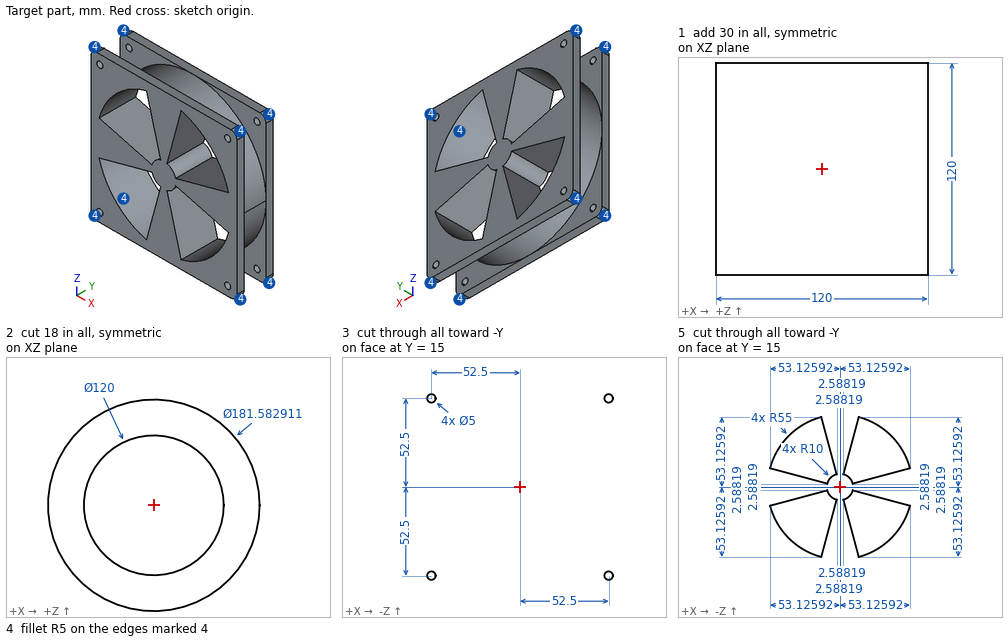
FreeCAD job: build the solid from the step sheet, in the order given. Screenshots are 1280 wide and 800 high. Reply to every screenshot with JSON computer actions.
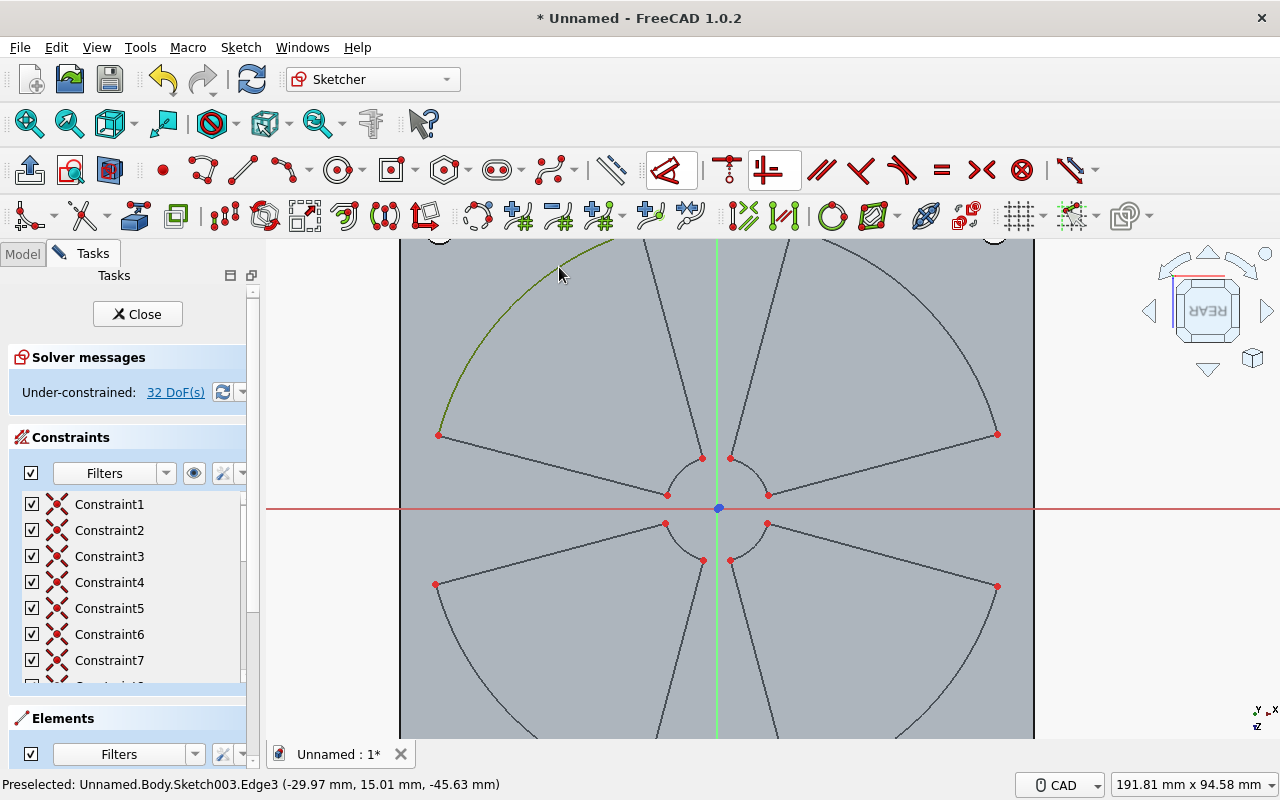
{"action": "left_click", "coordinate": [745, 554]}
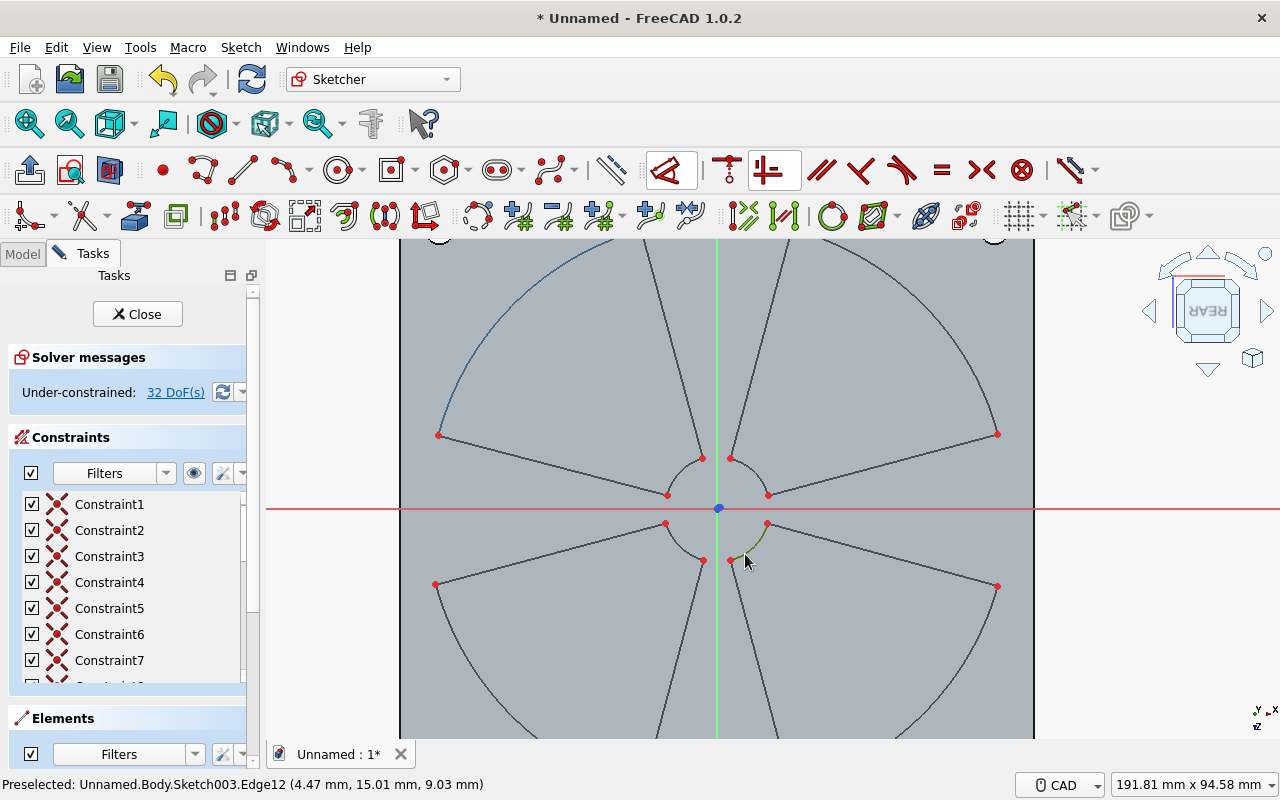
{"action": "left_click", "coordinate": [728, 170]}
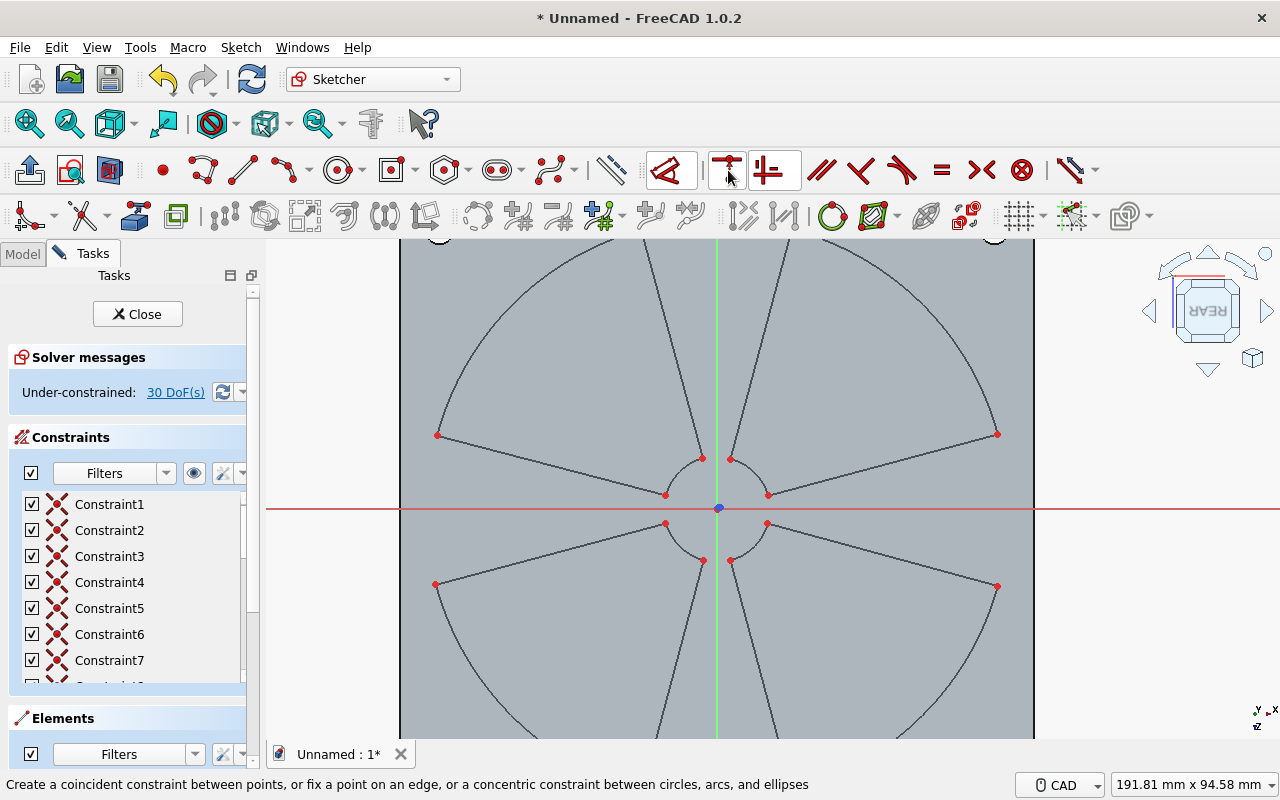
{"action": "left_click", "coordinate": [559, 267]}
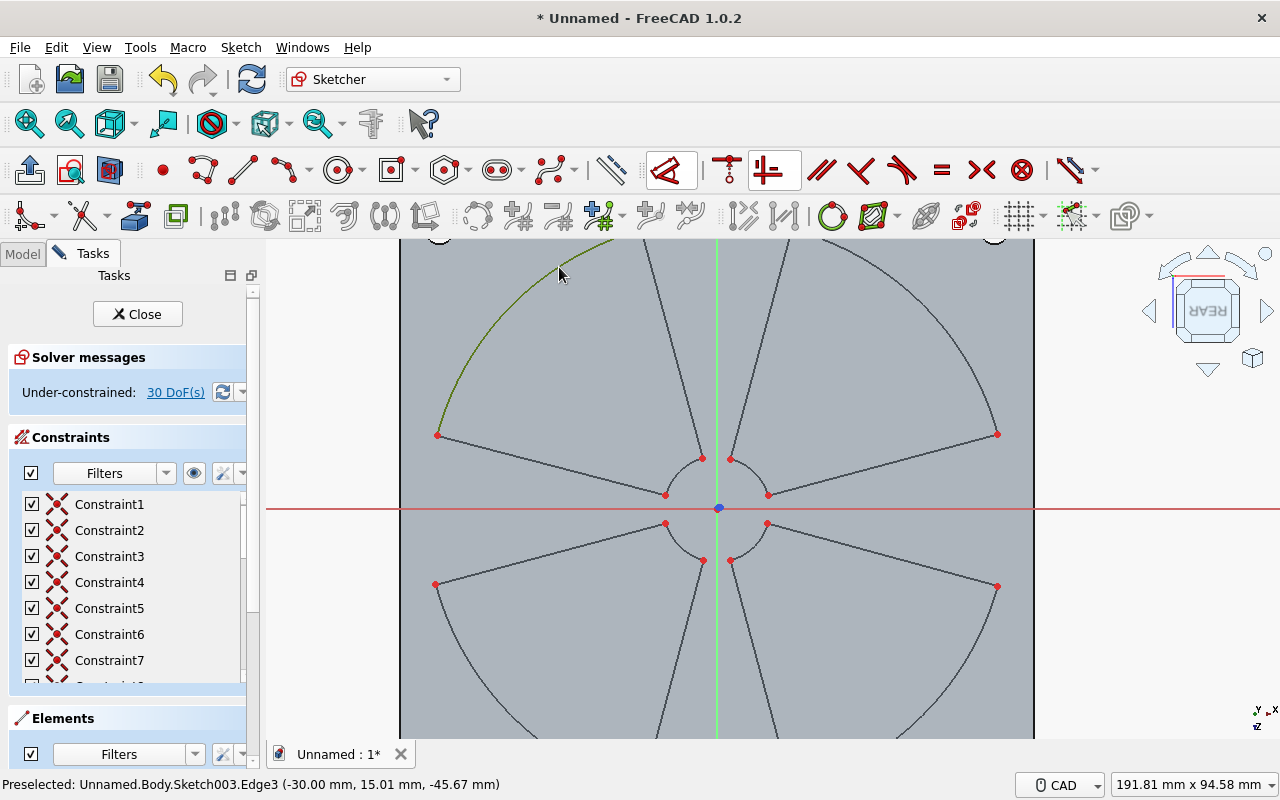
{"action": "left_click", "coordinate": [673, 538]}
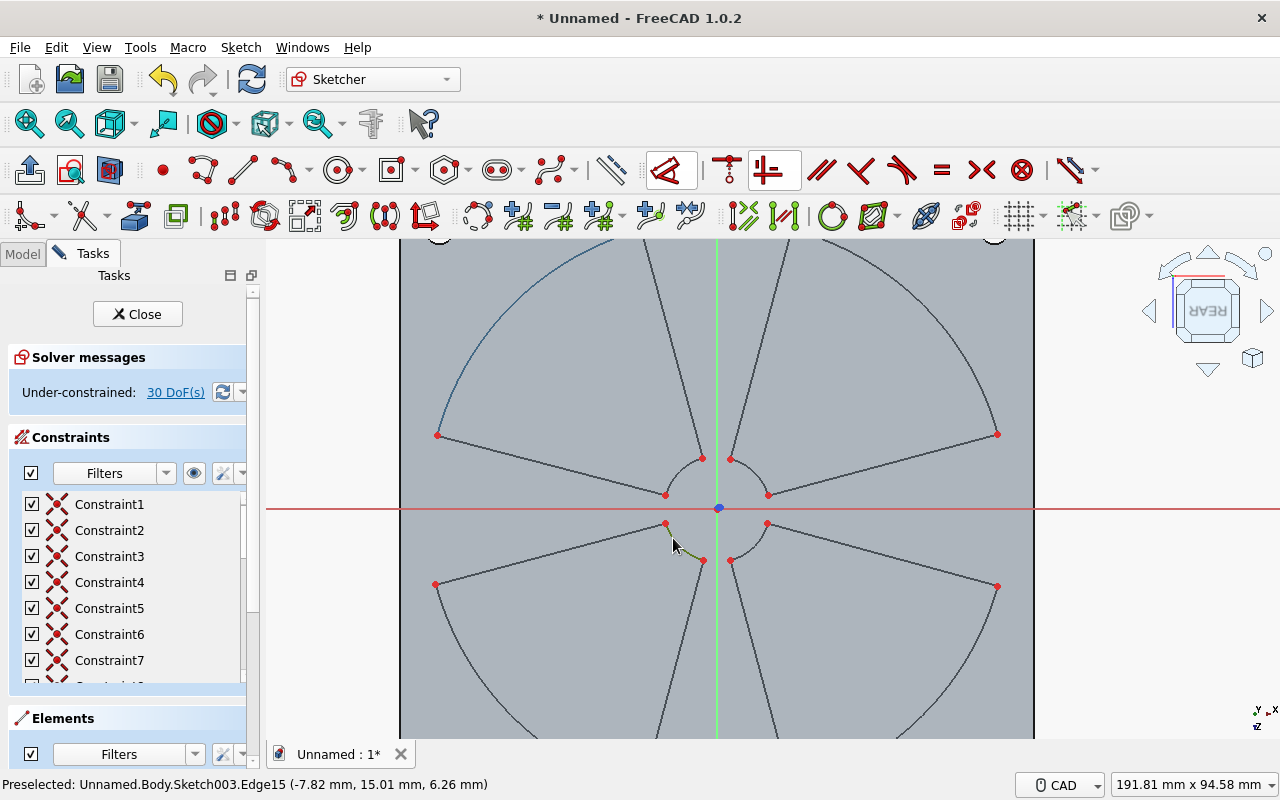
{"action": "left_click", "coordinate": [728, 170]}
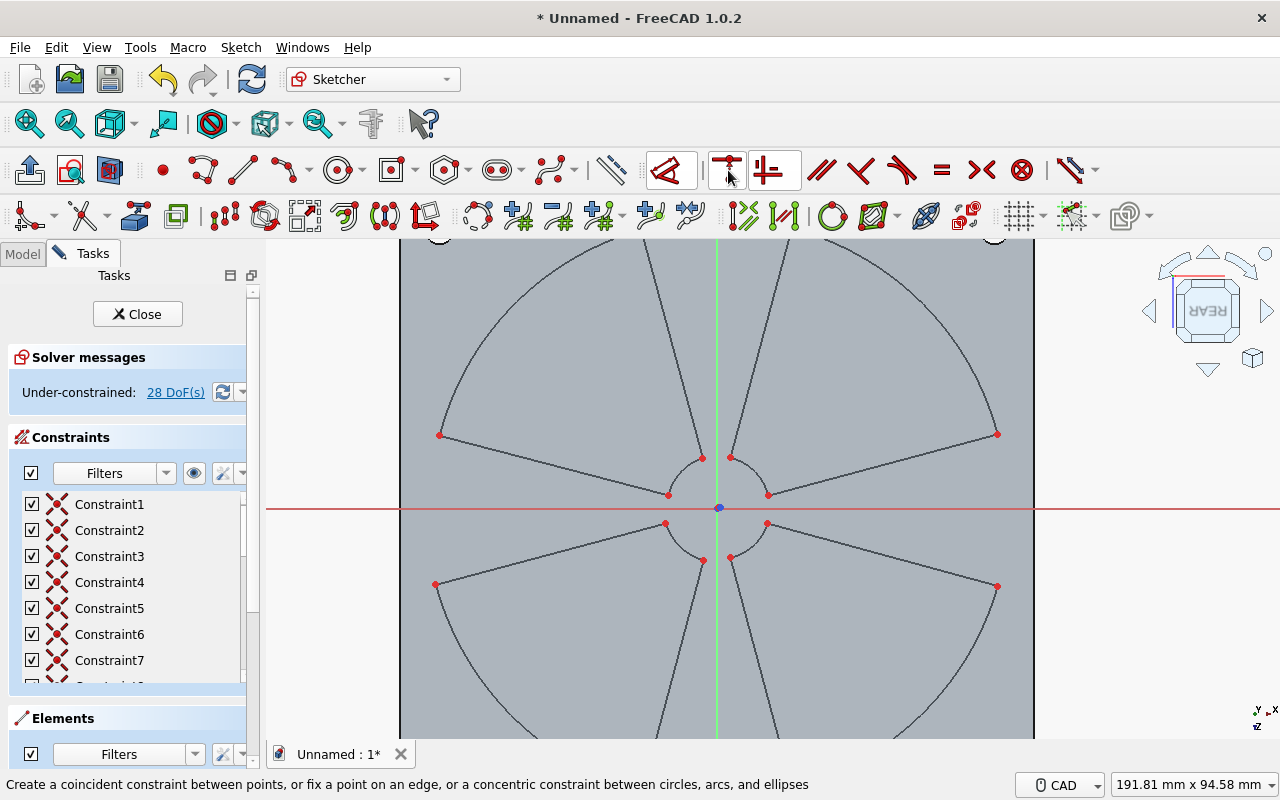
{"action": "left_click", "coordinate": [559, 267]}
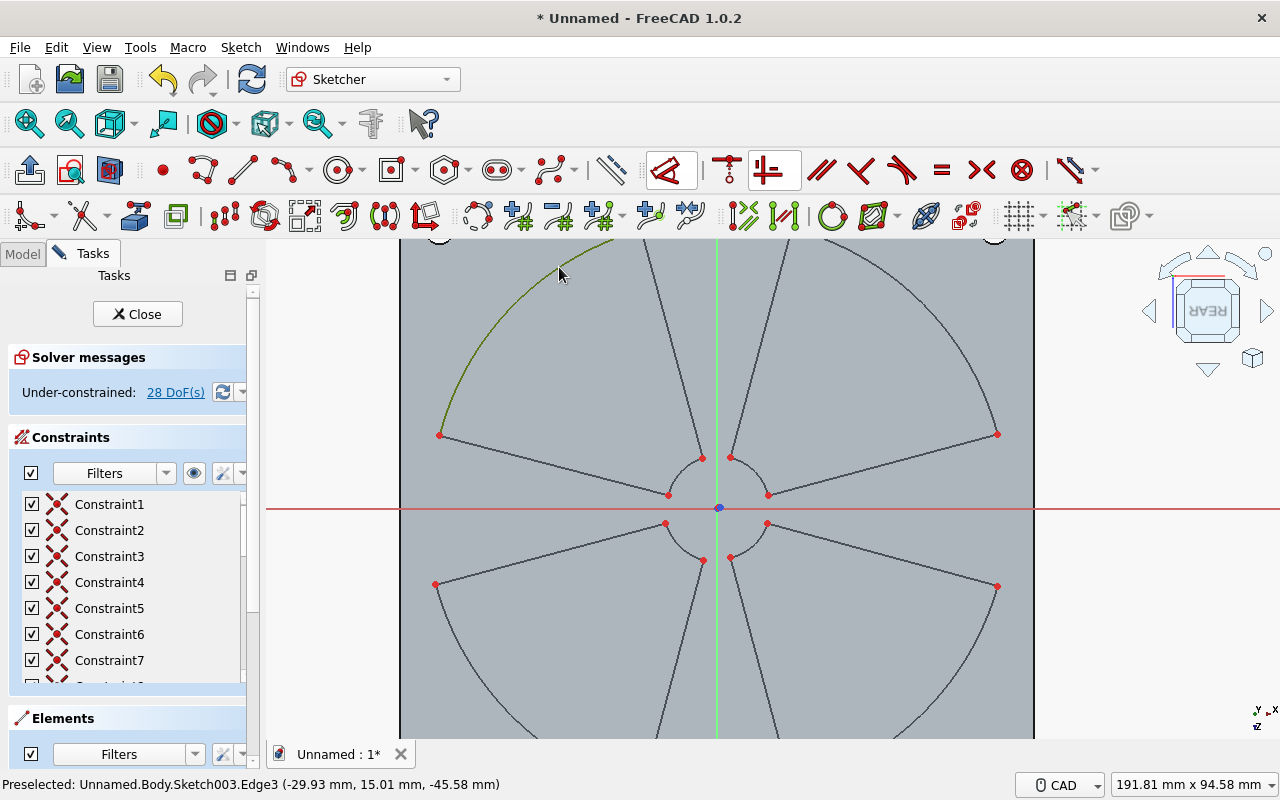
{"action": "left_click", "coordinate": [473, 668]}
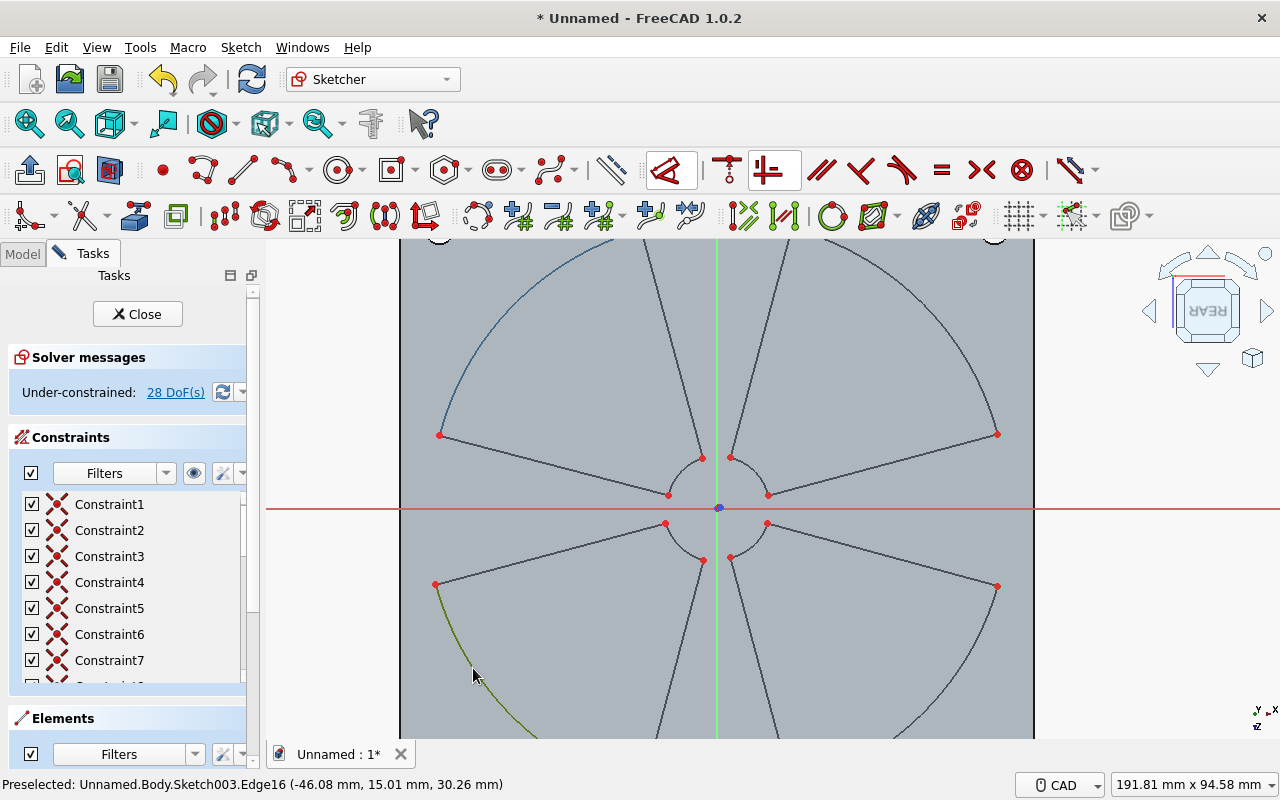
{"action": "left_click", "coordinate": [728, 170]}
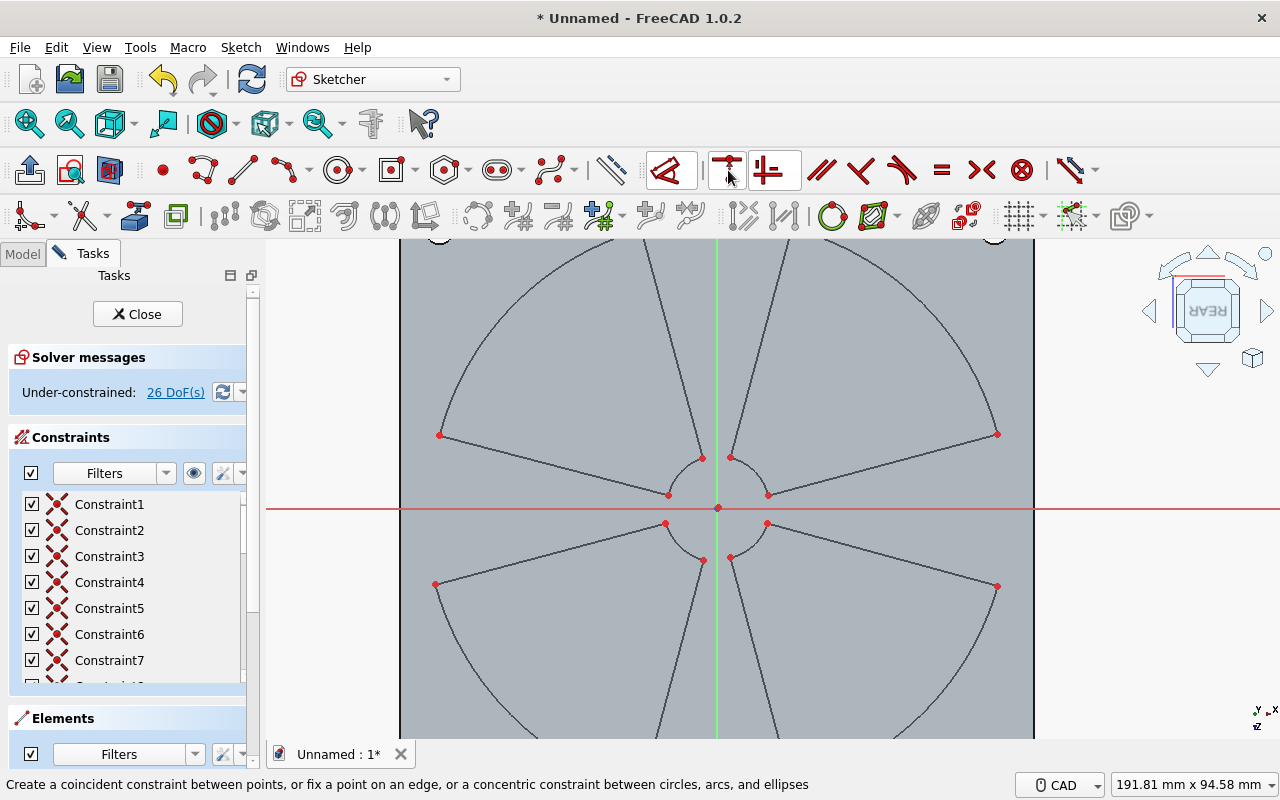
{"action": "left_click_drag", "start_coordinate": [707, 497], "coordinate": [729, 519]}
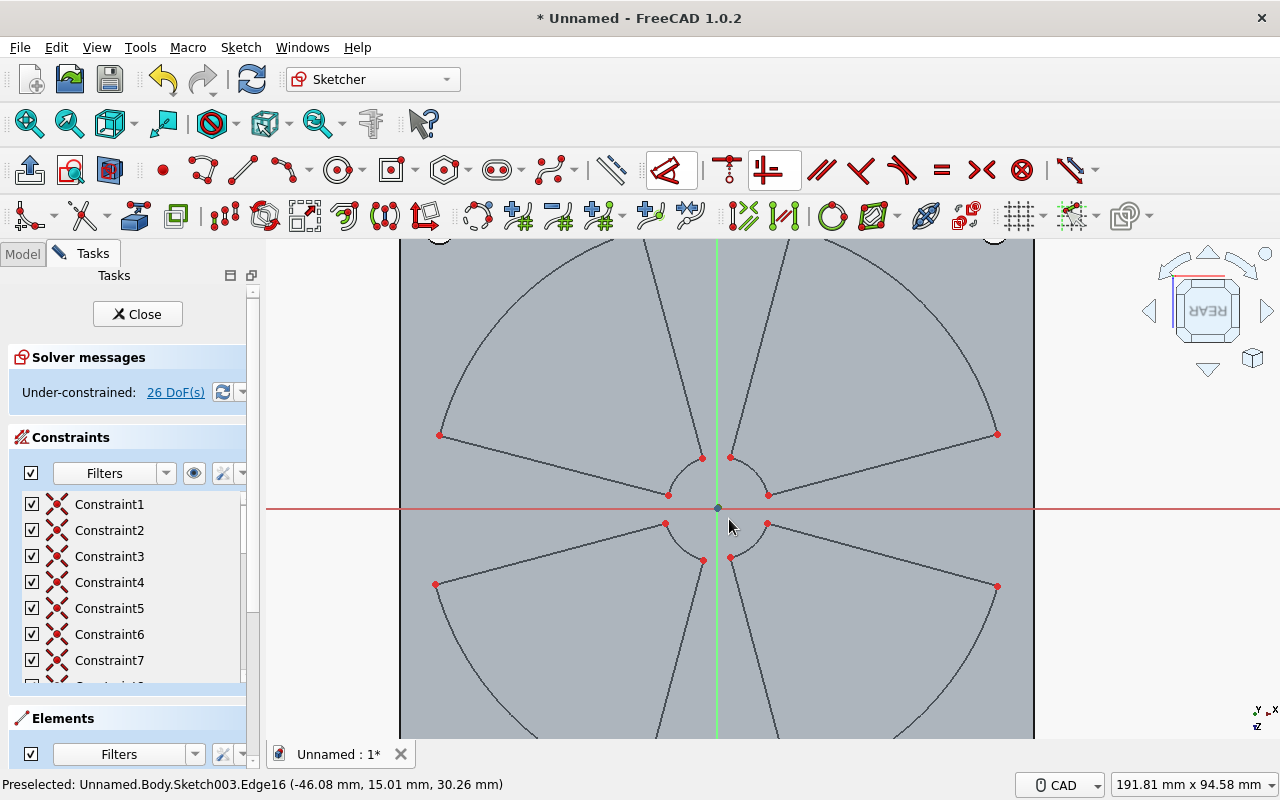
{"action": "left_click", "coordinate": [728, 170]}